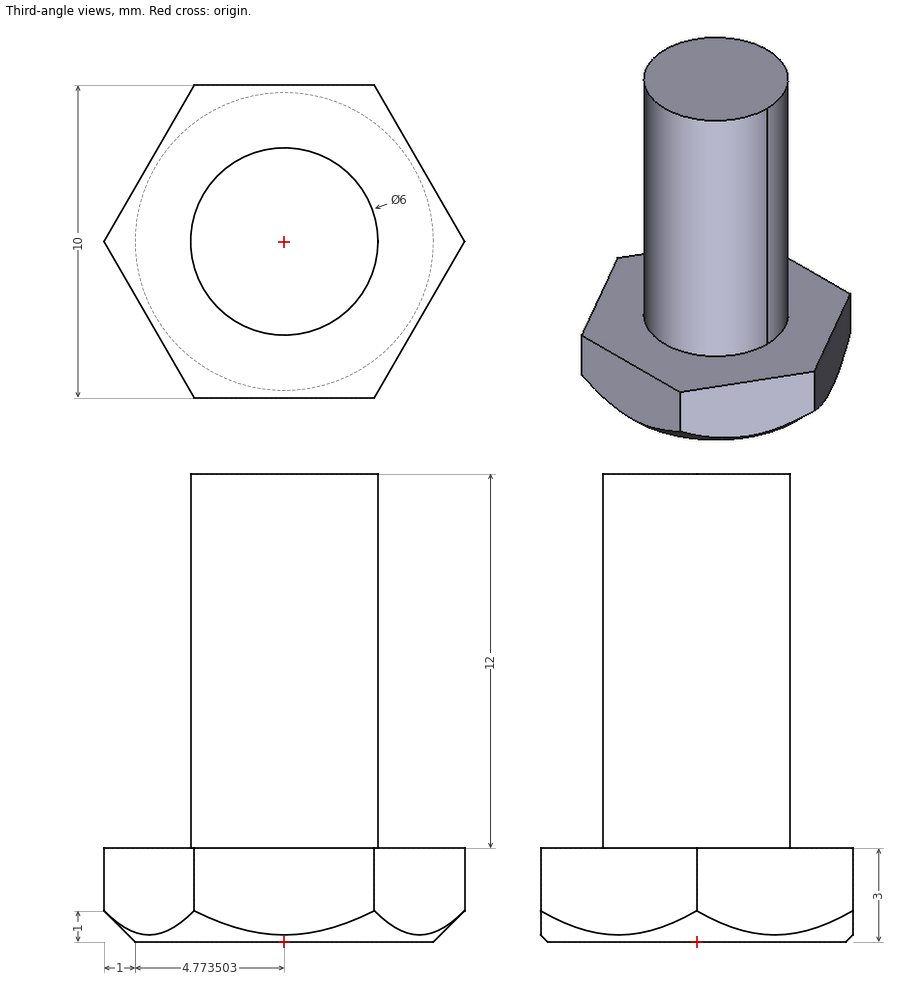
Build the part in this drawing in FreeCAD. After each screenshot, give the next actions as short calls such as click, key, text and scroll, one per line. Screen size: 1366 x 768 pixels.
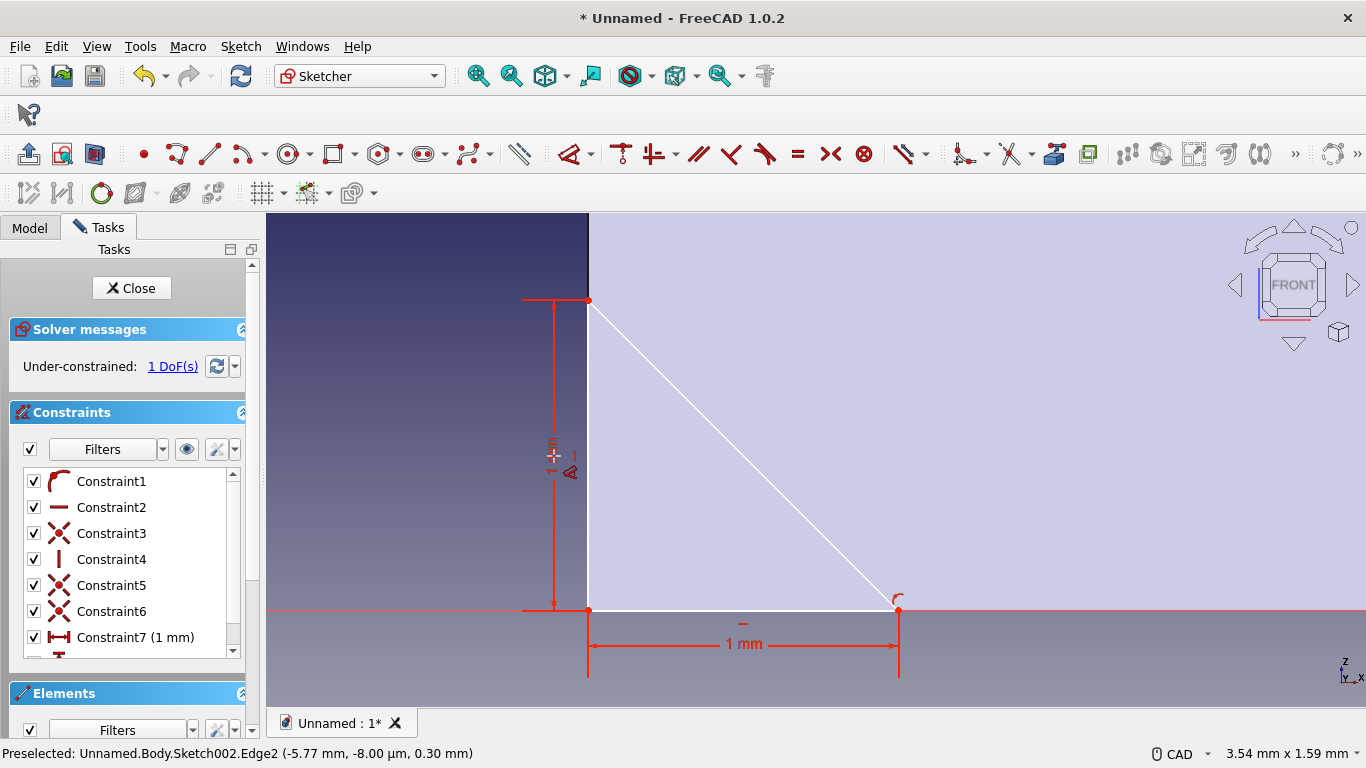
click(899, 611)
click(1050, 645)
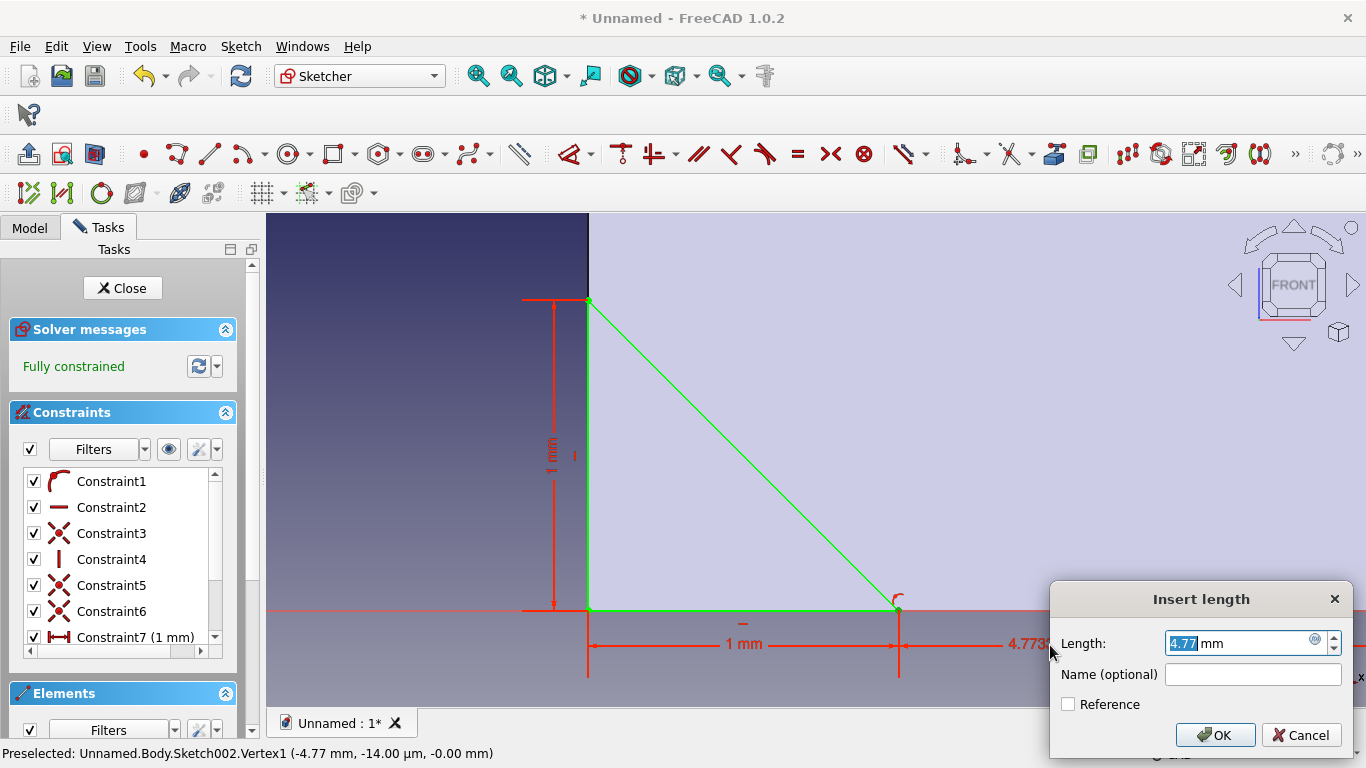
text(4.773503)
key(Return)
key(Escape)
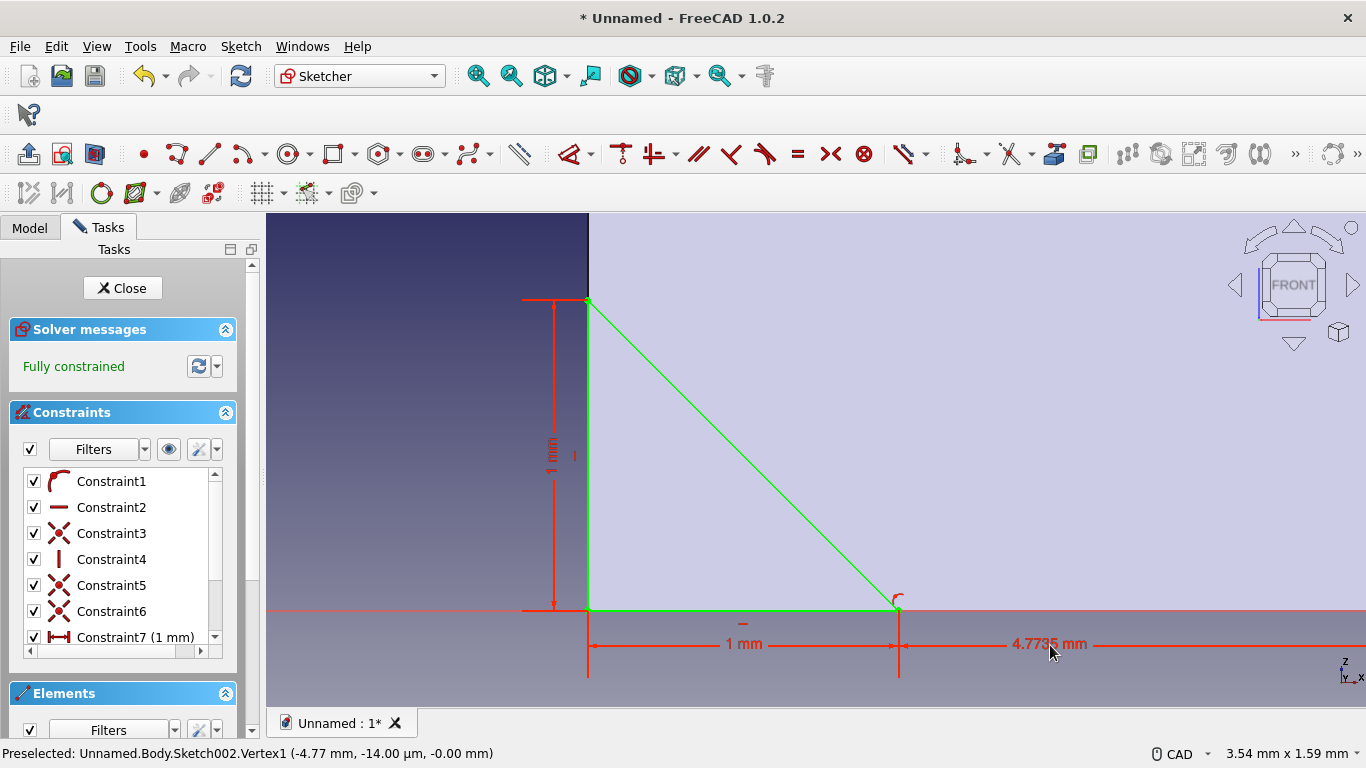
click(123, 288)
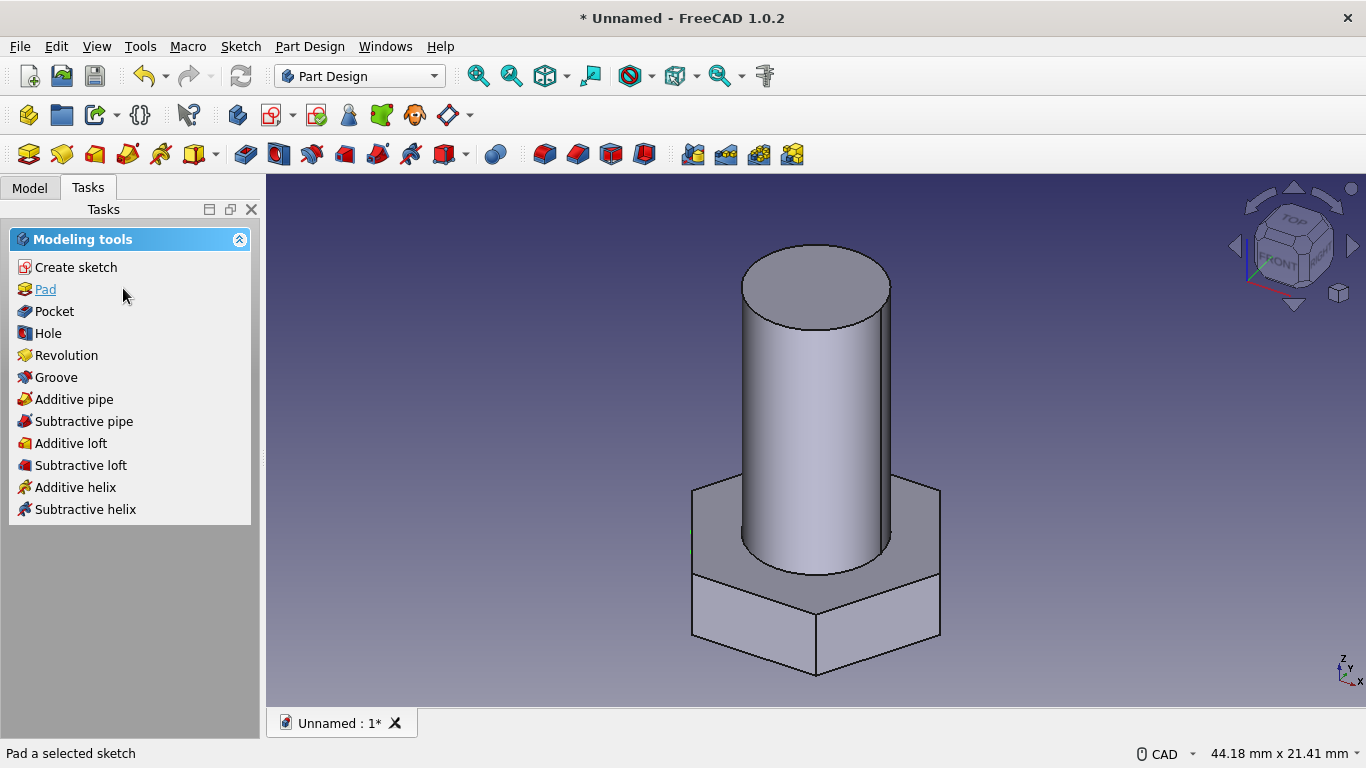
click(312, 154)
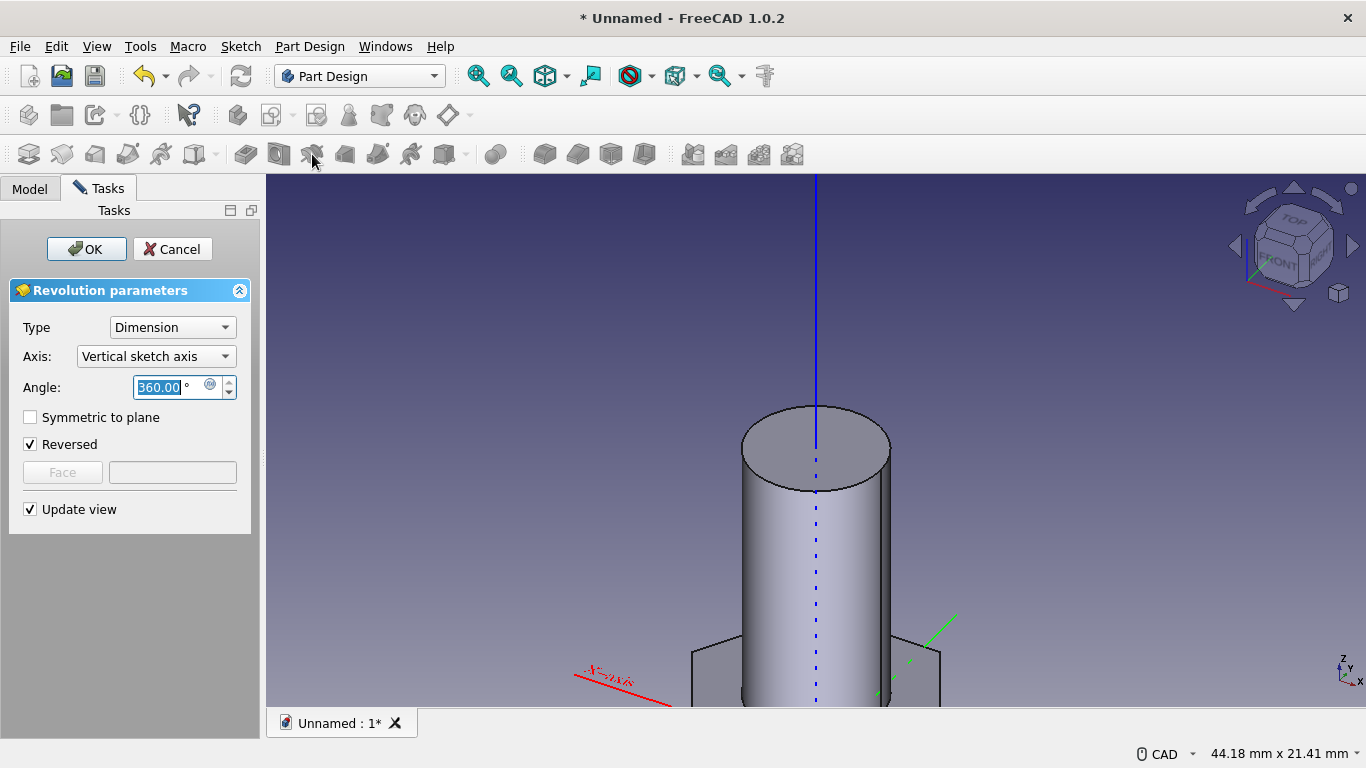
click(87, 249)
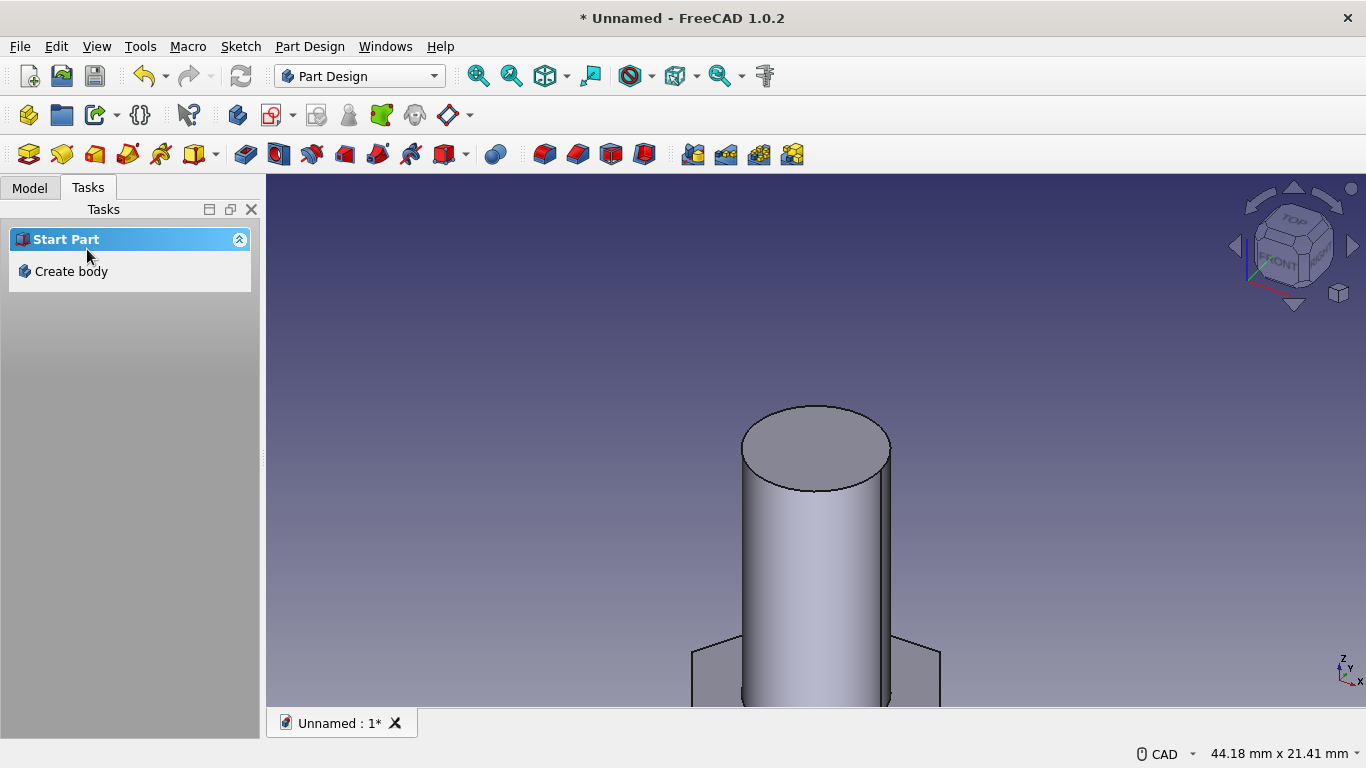
key(0)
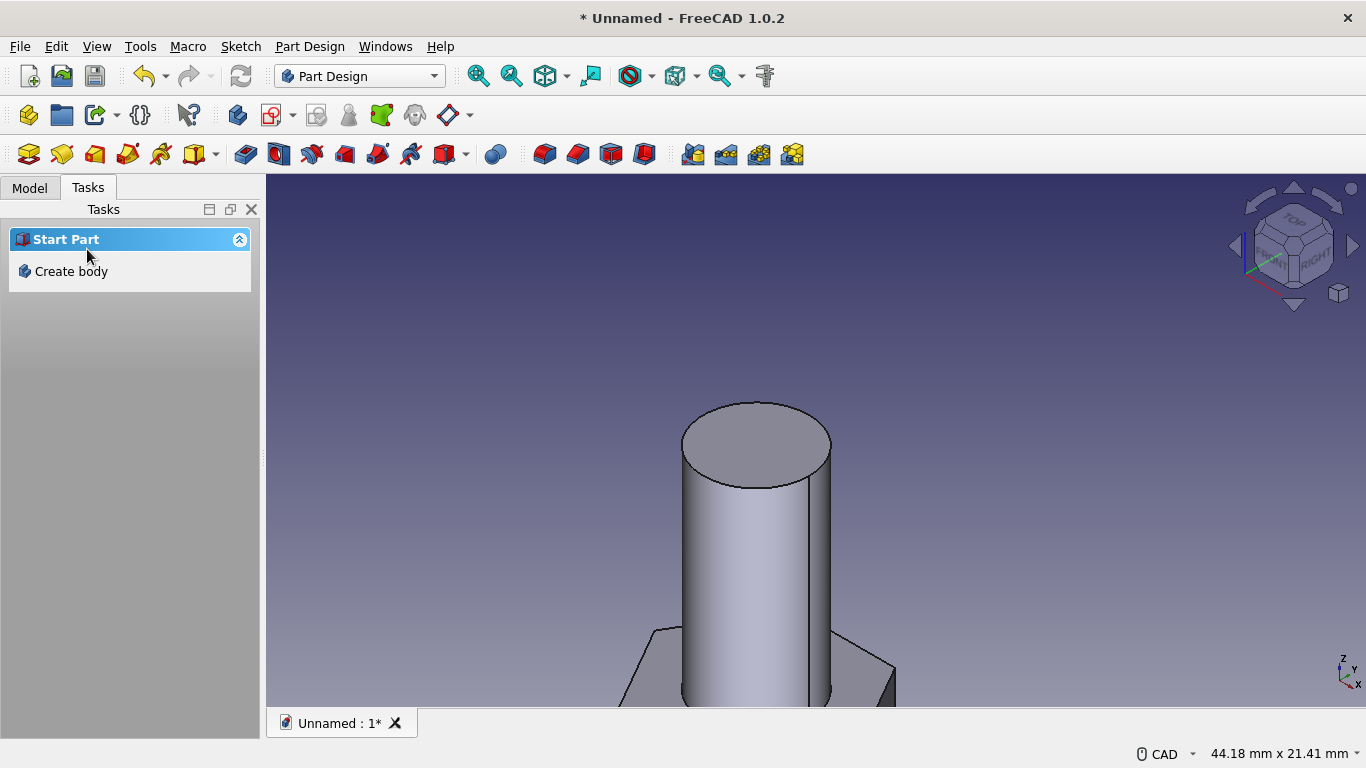
click(479, 76)